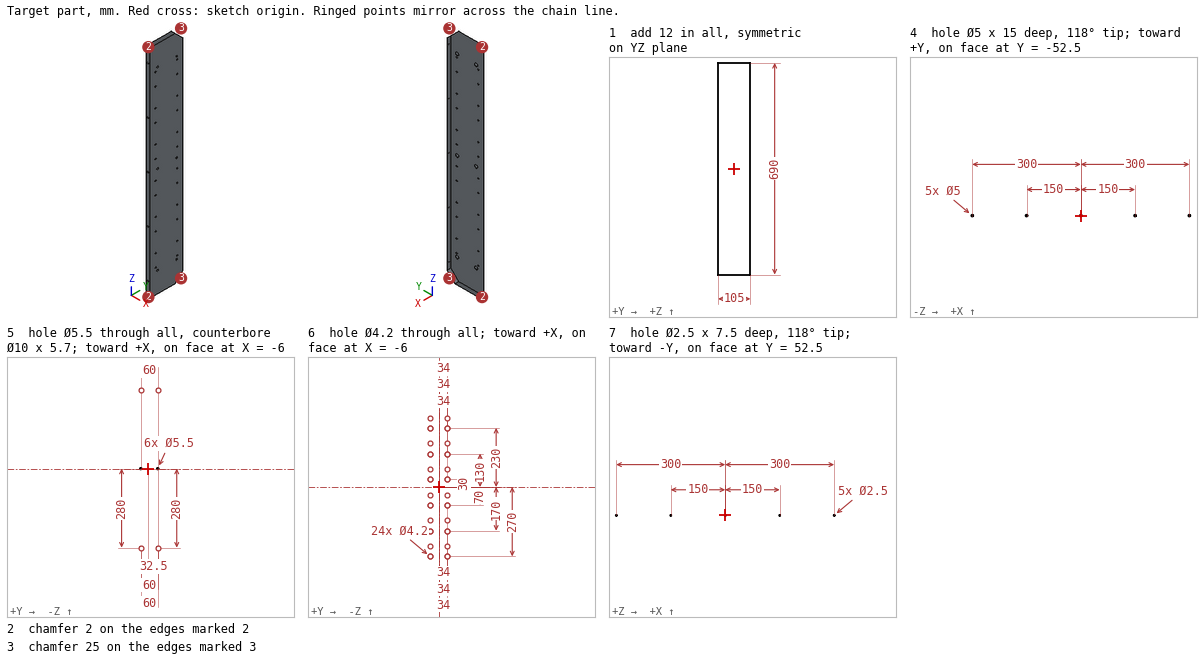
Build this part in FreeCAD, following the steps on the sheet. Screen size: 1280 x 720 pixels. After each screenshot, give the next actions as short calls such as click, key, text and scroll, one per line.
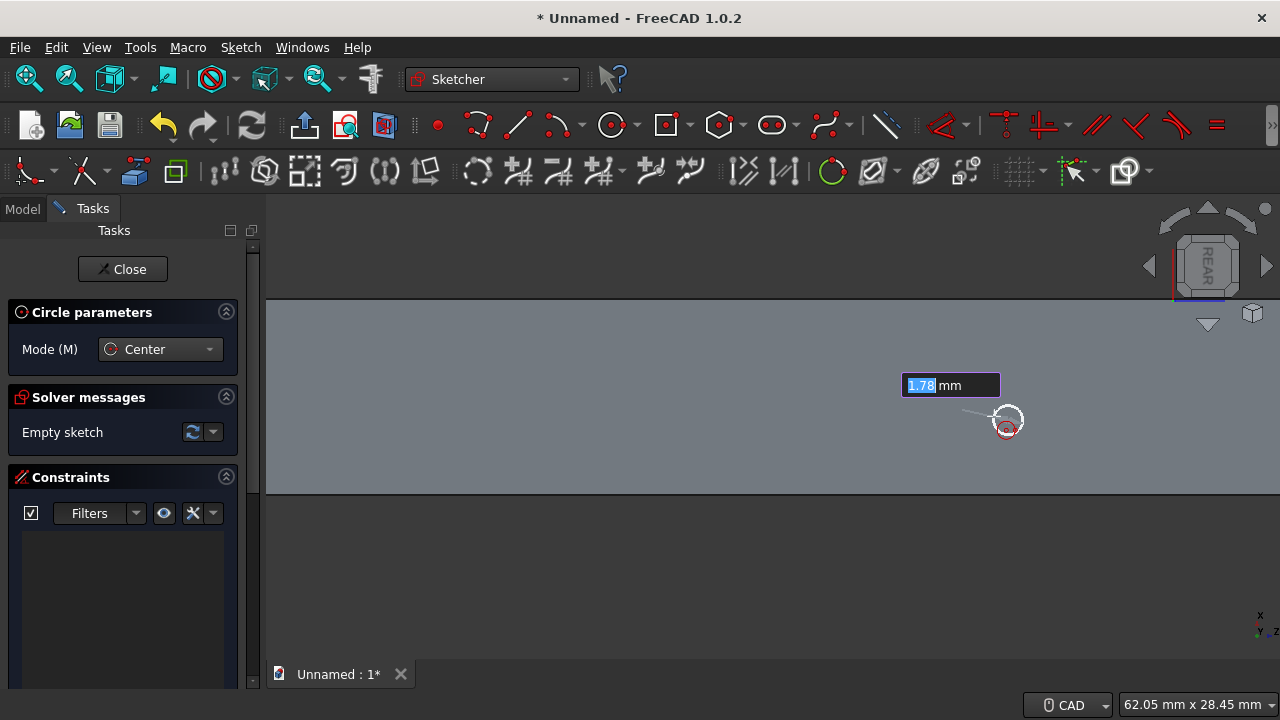
text(2.5)
key(Return)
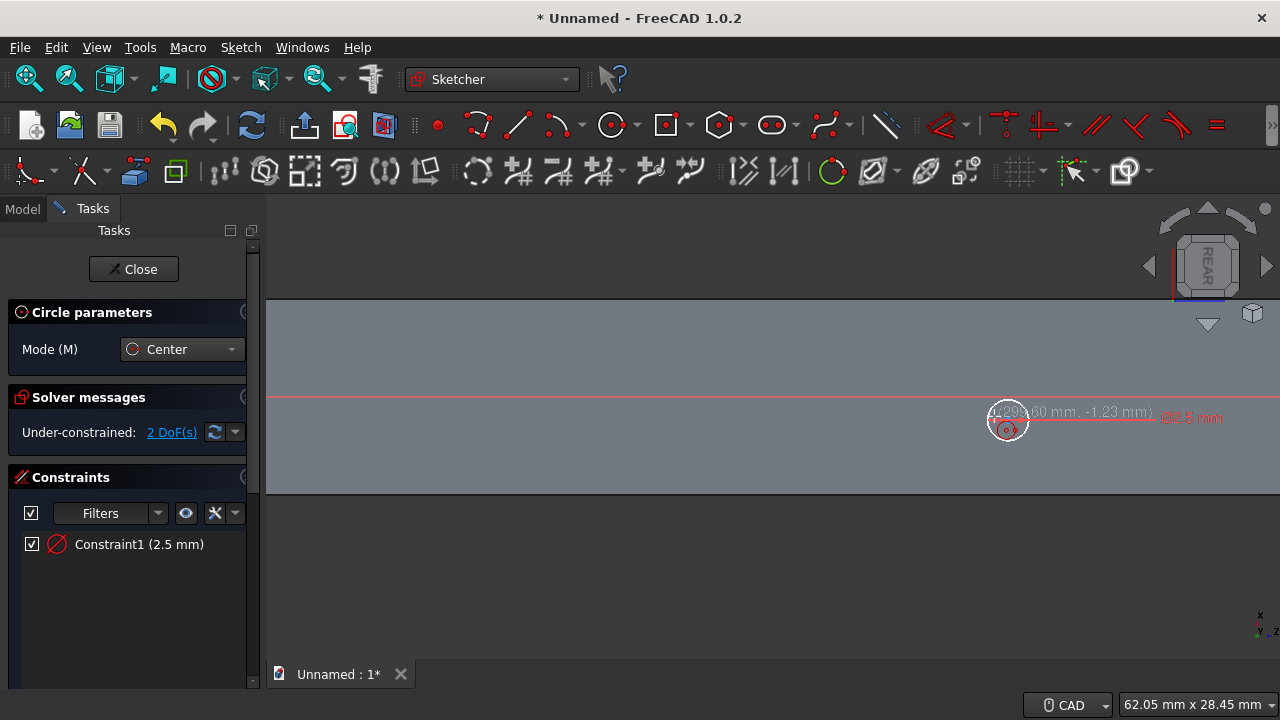
scroll(1003, 428, down, 14)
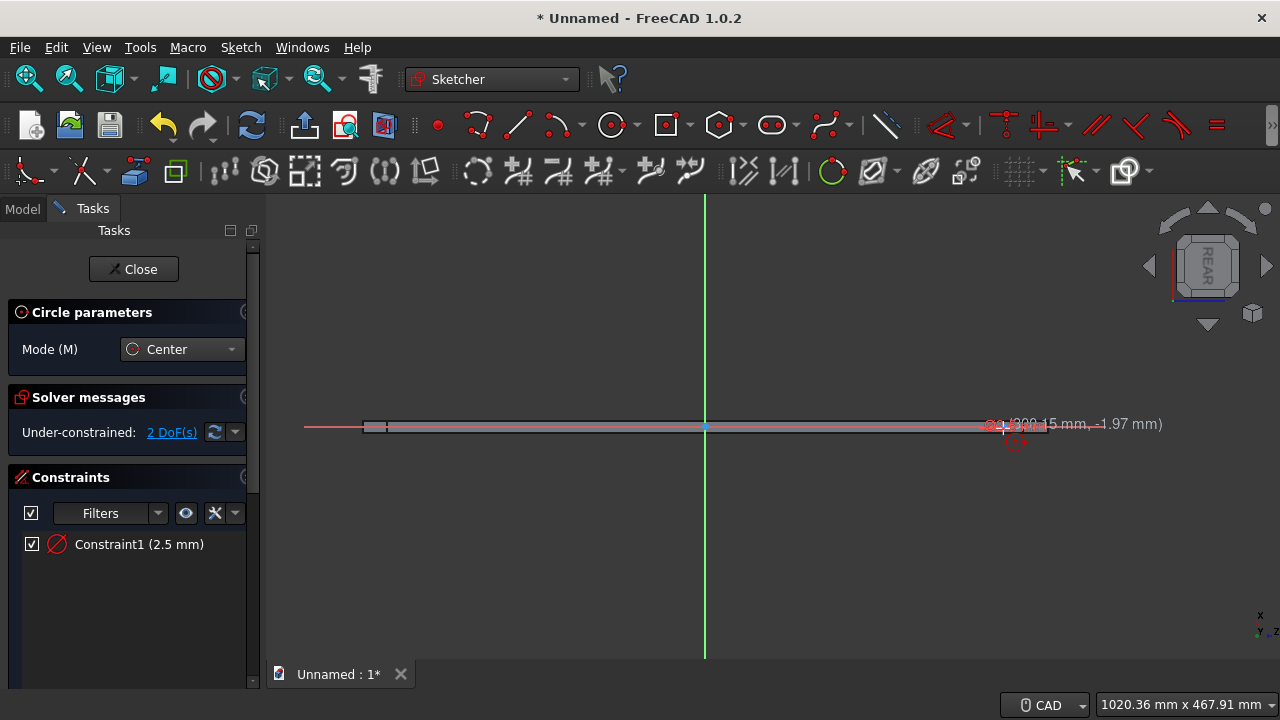
scroll(854, 427, up, 15)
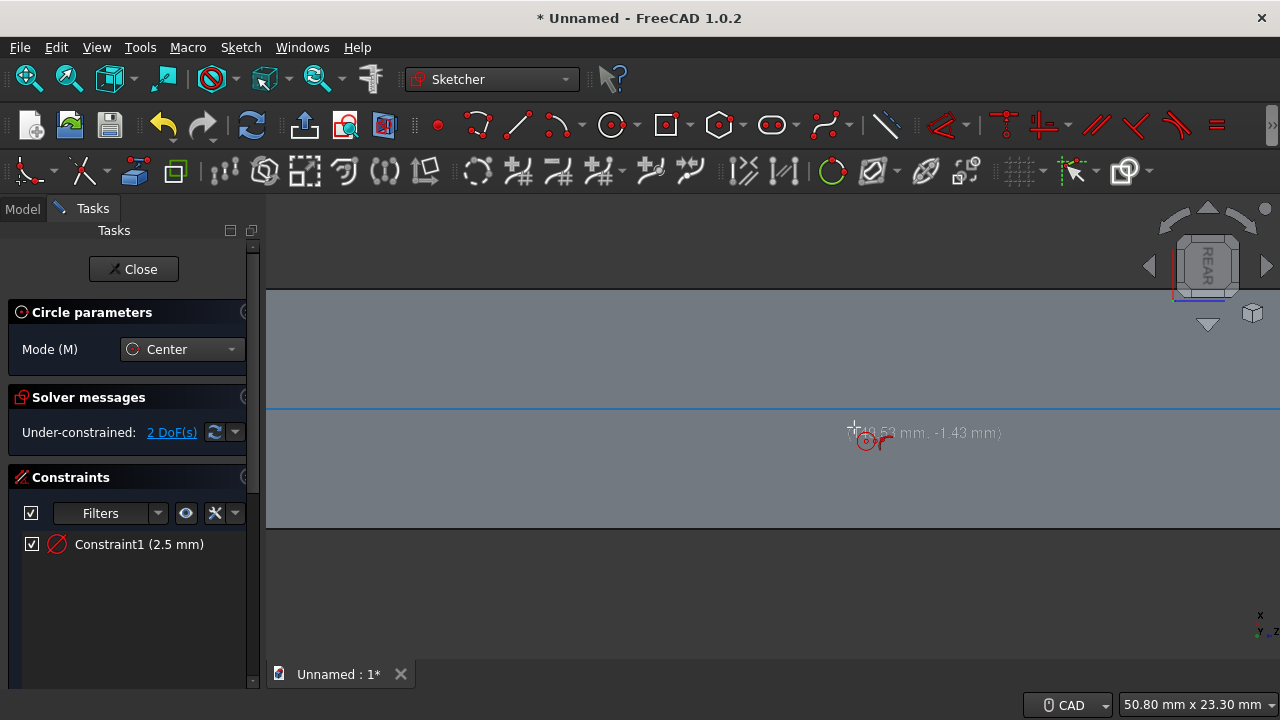
scroll(854, 427, down, 15)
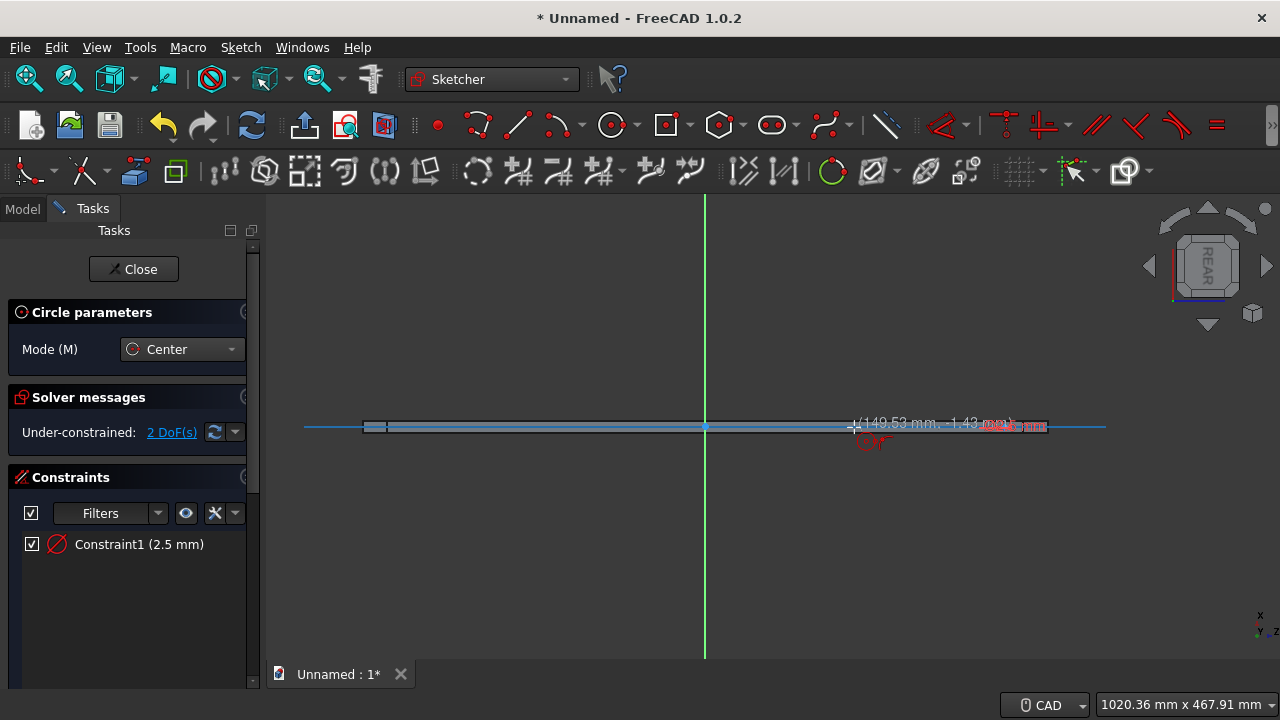
click(854, 427)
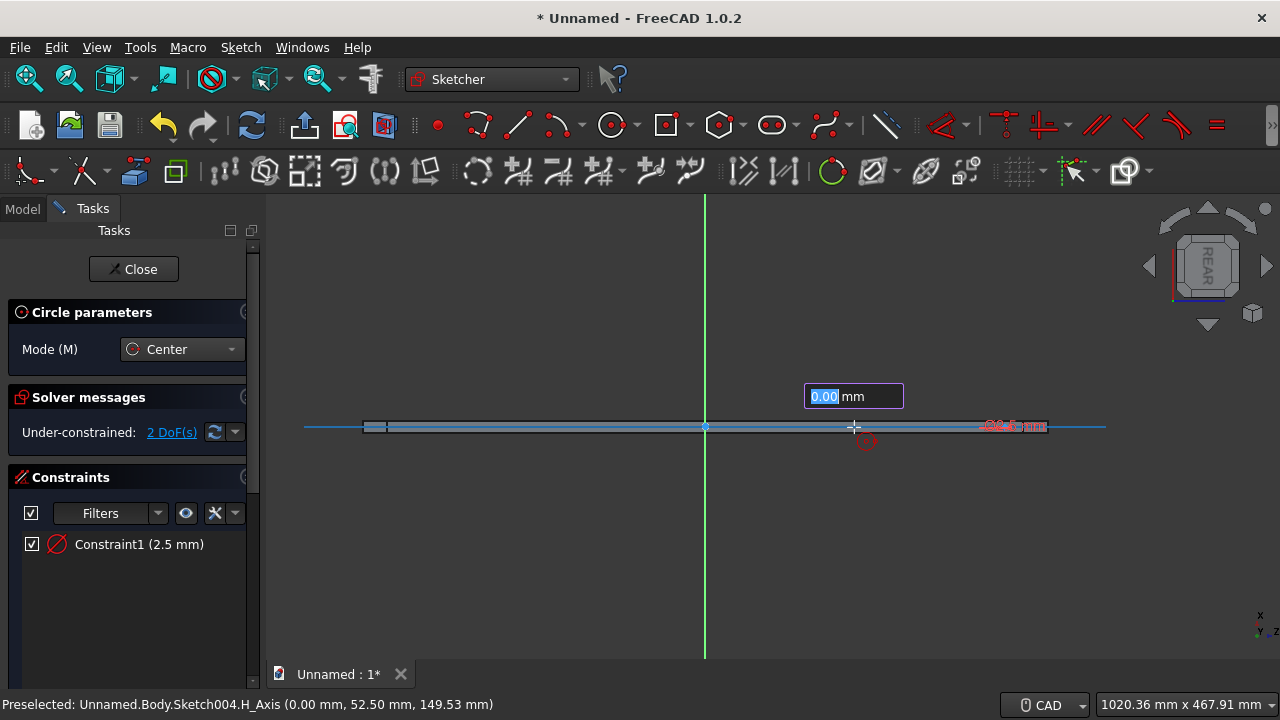
scroll(854, 428, up, 14)
move(846, 416)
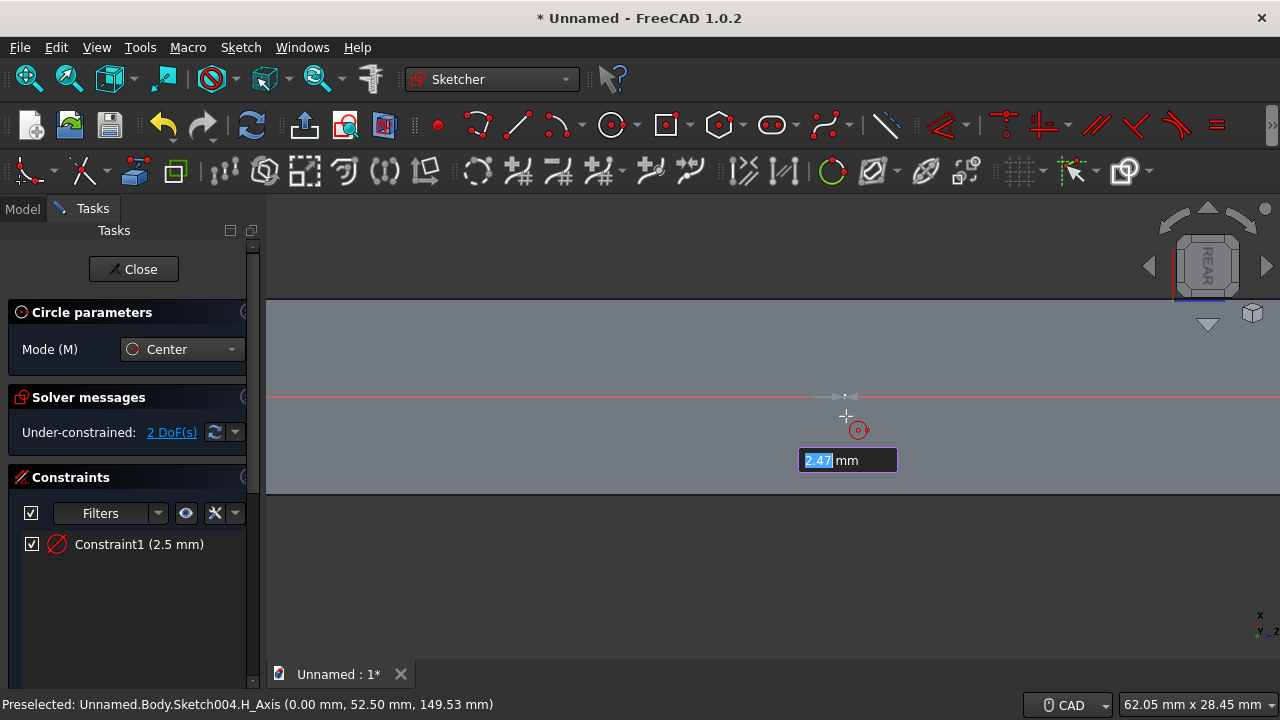
text(2.5)
key(Return)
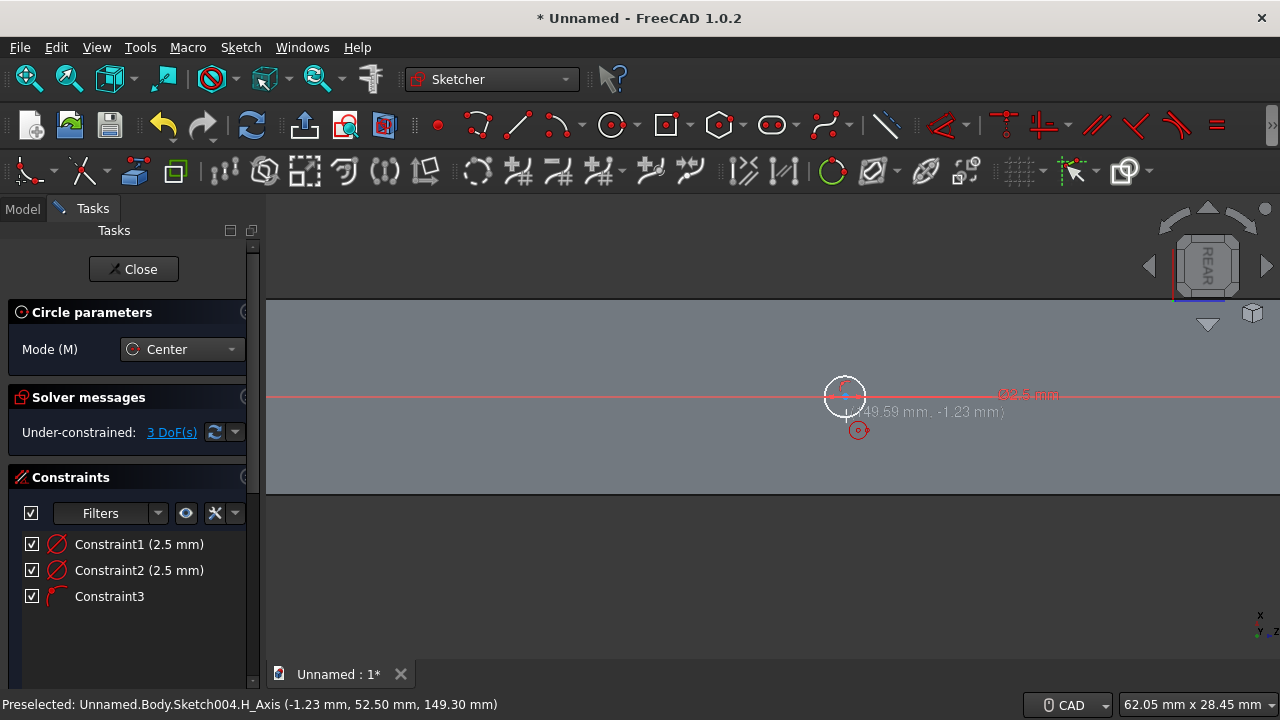
scroll(854, 428, down, 14)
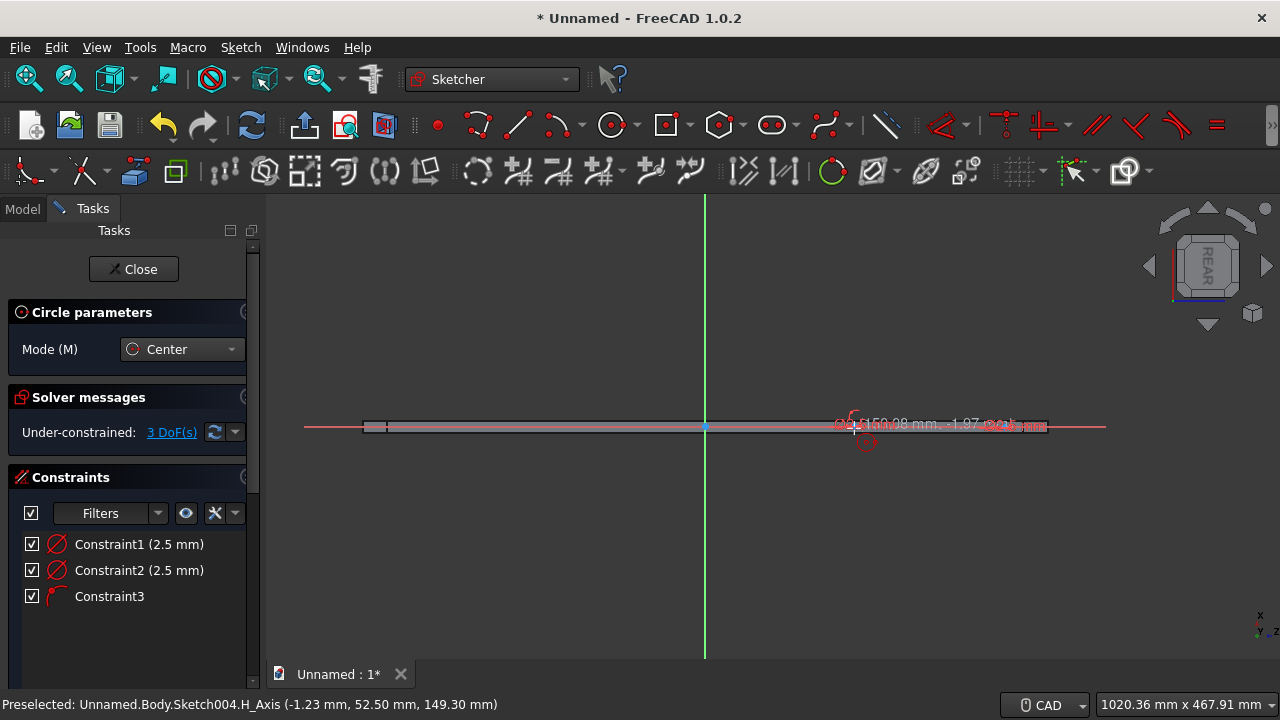
scroll(705, 427, up, 15)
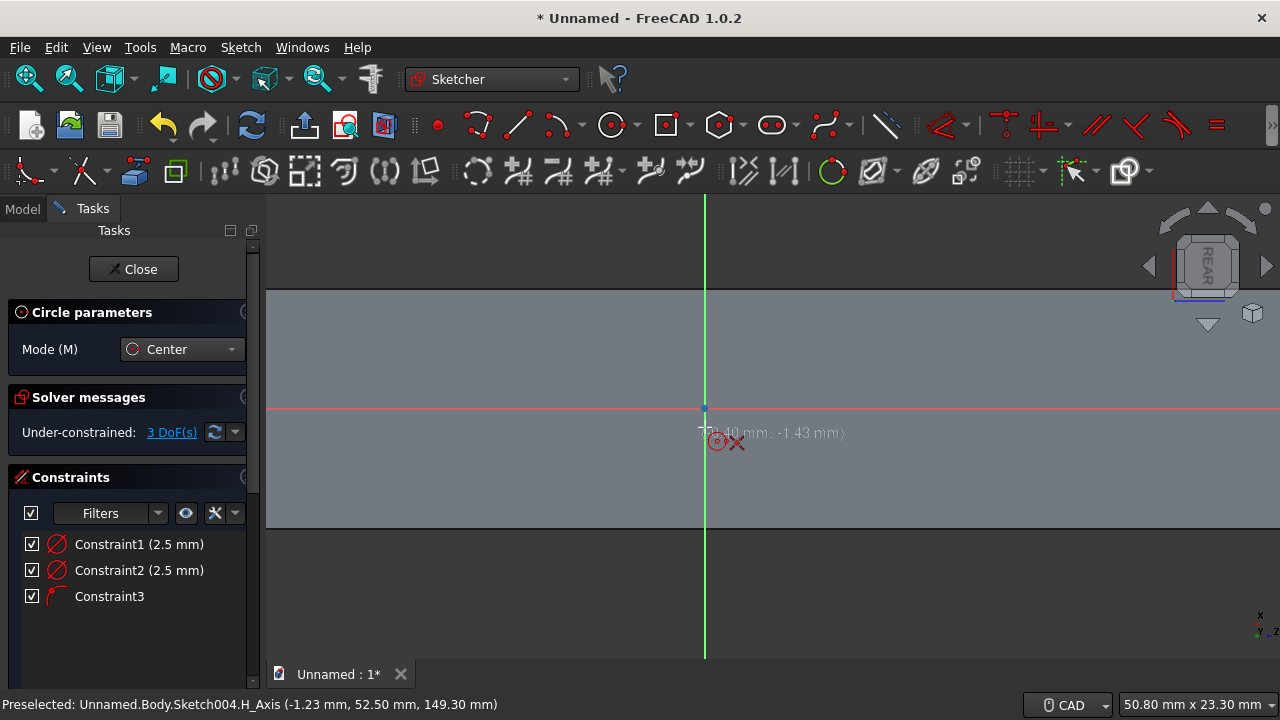
scroll(704, 427, down, 15)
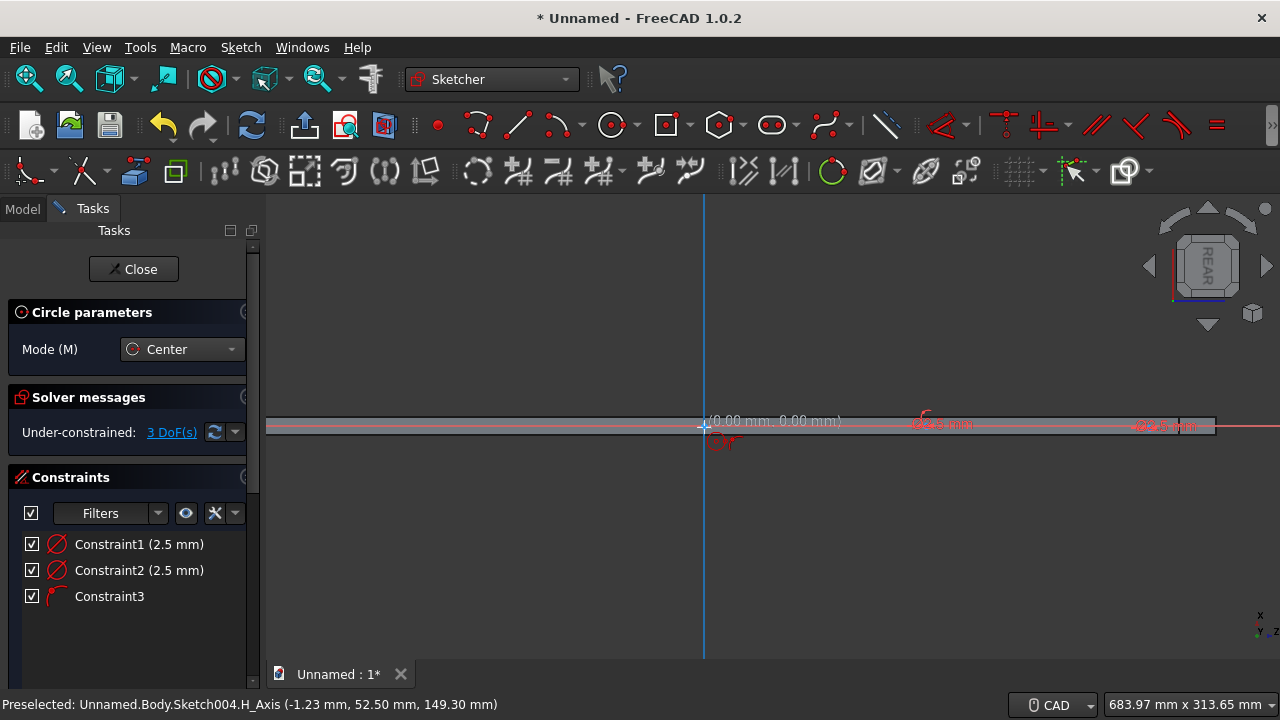
click(704, 427)